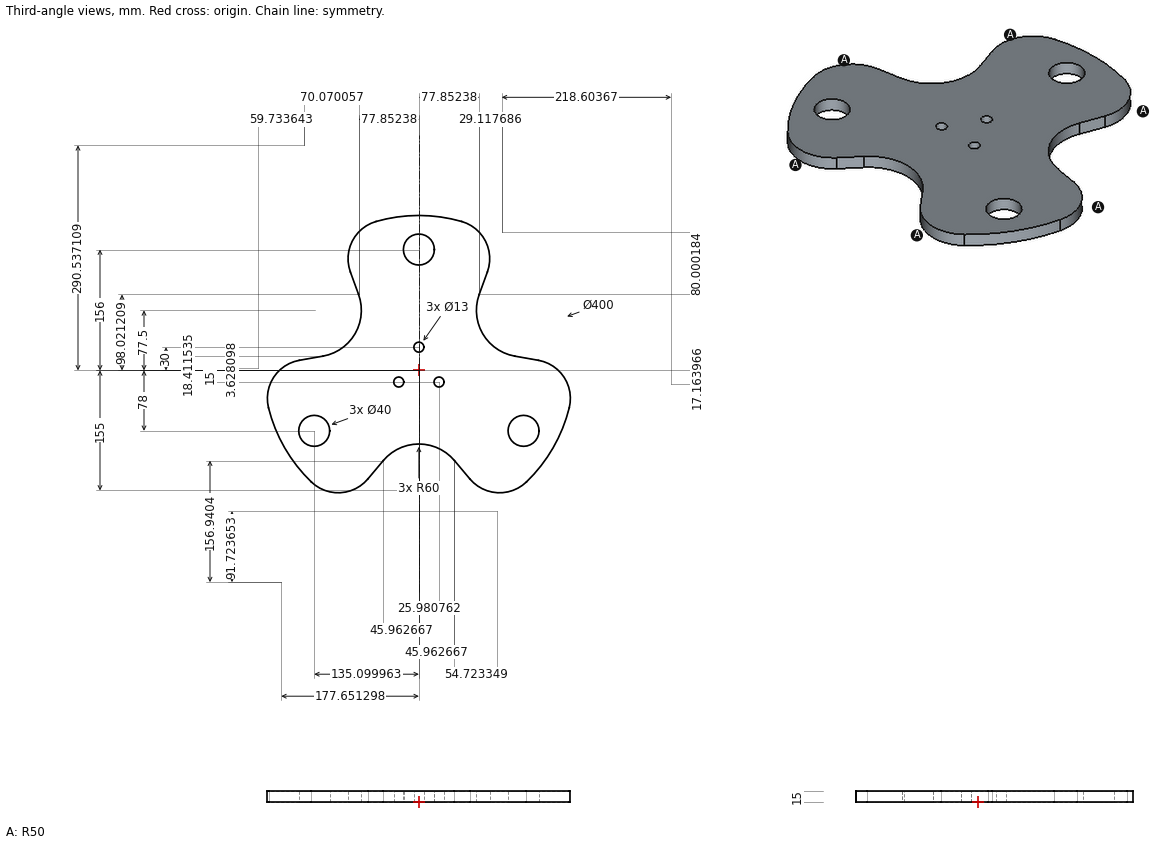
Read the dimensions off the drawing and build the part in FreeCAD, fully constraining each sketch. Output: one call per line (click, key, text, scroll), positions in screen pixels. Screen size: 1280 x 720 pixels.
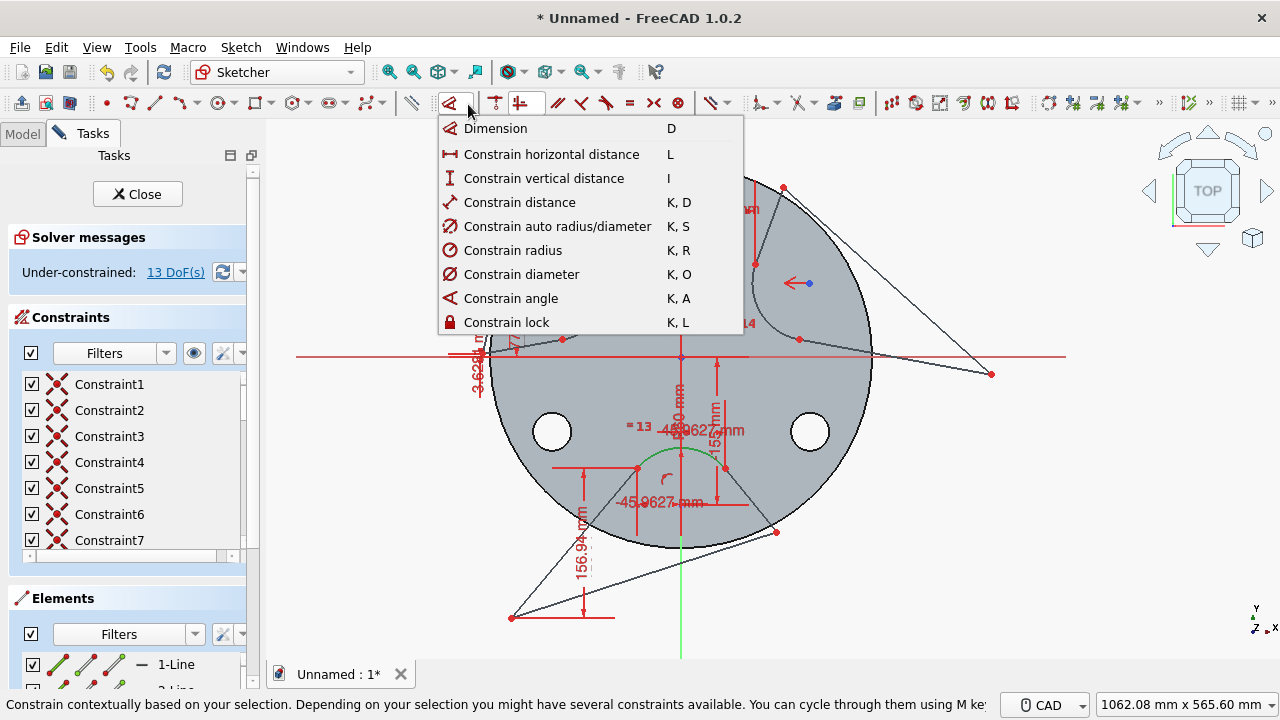
click(591, 178)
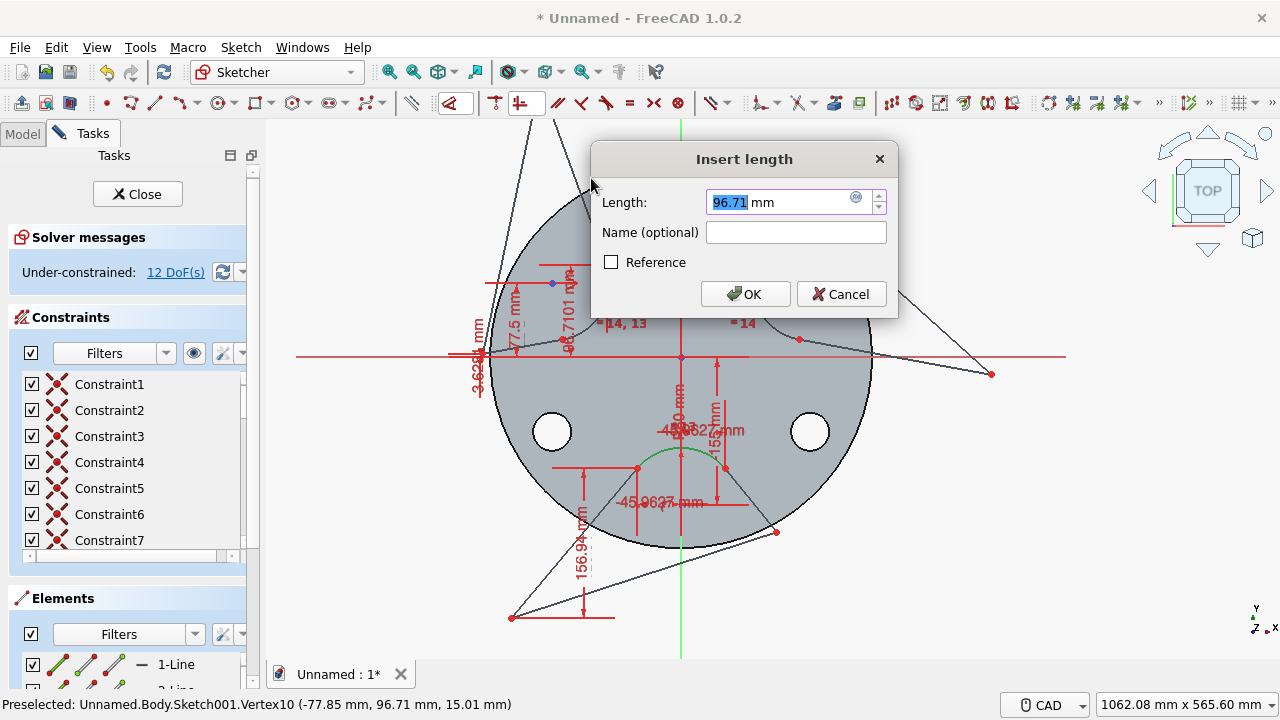
text(98.021209)
key(Return)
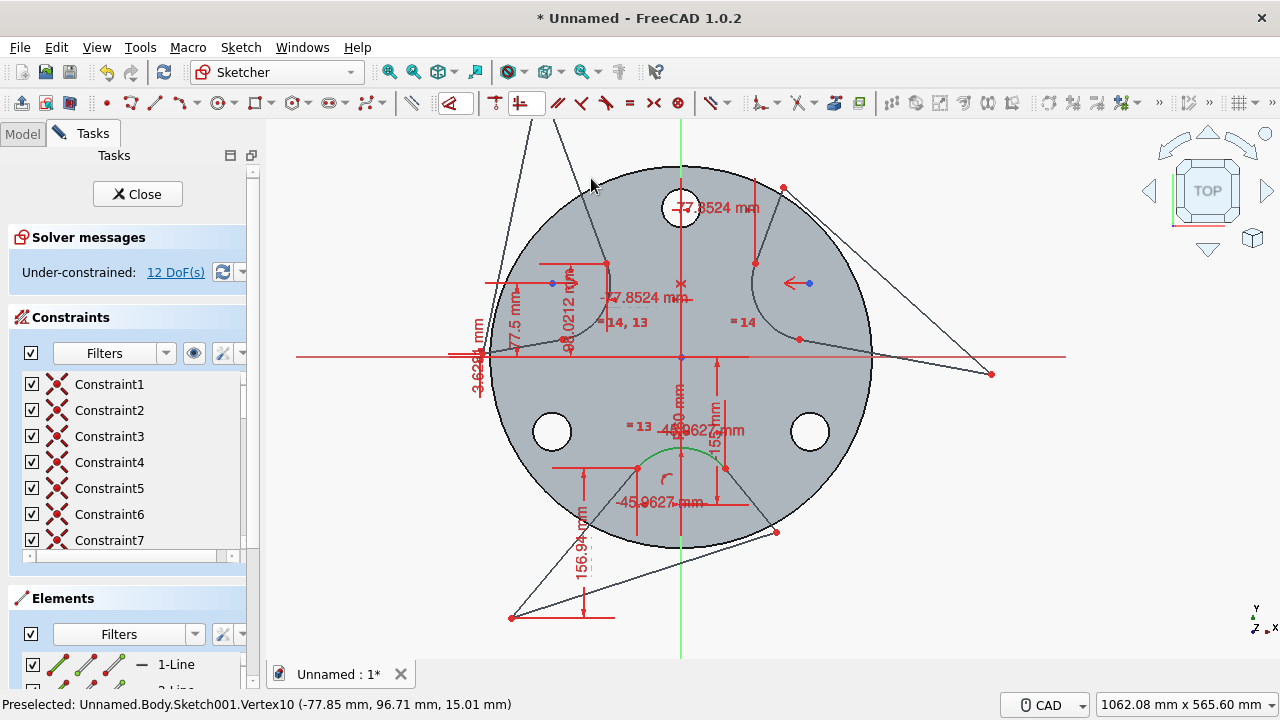
scroll(563, 340, up, 5)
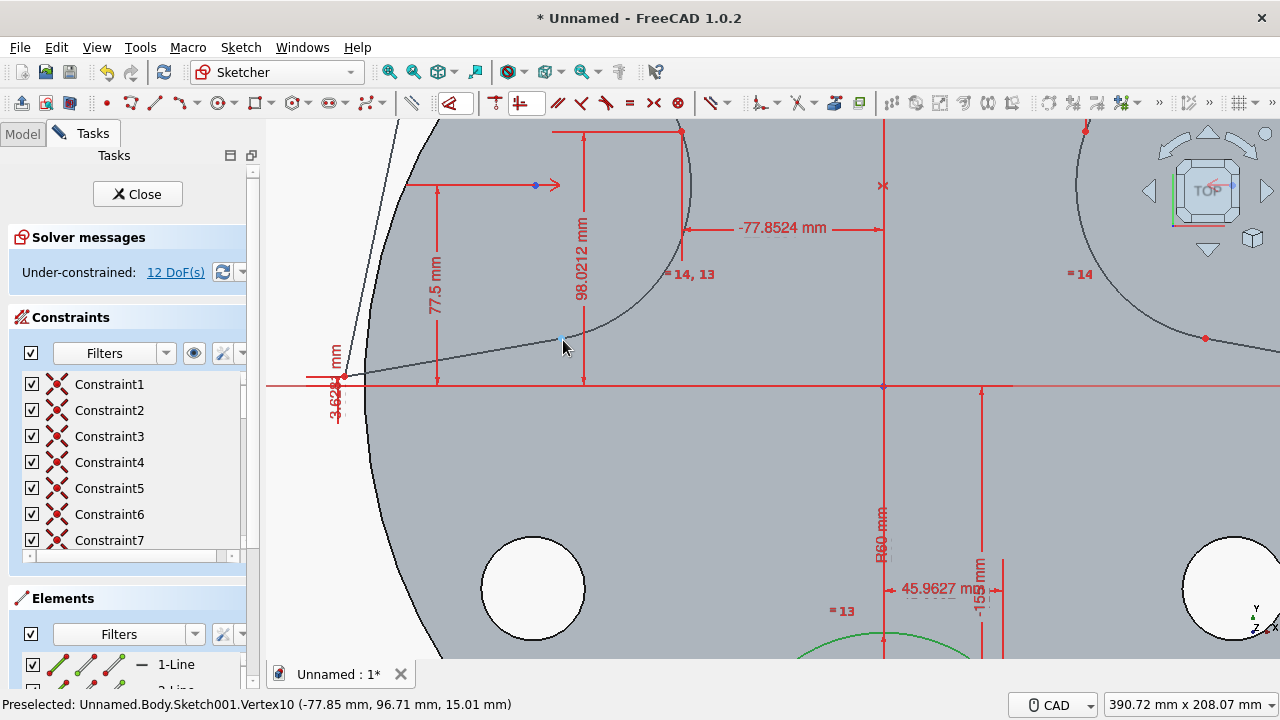
click(562, 339)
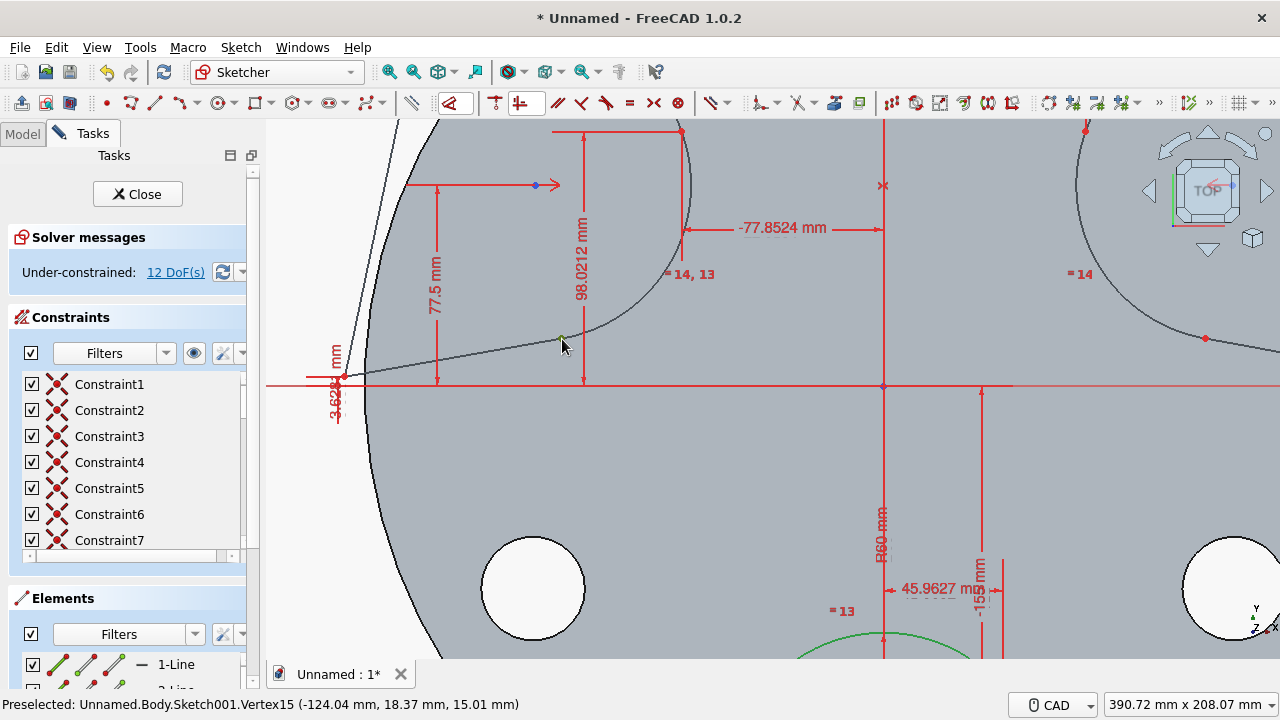
key(i)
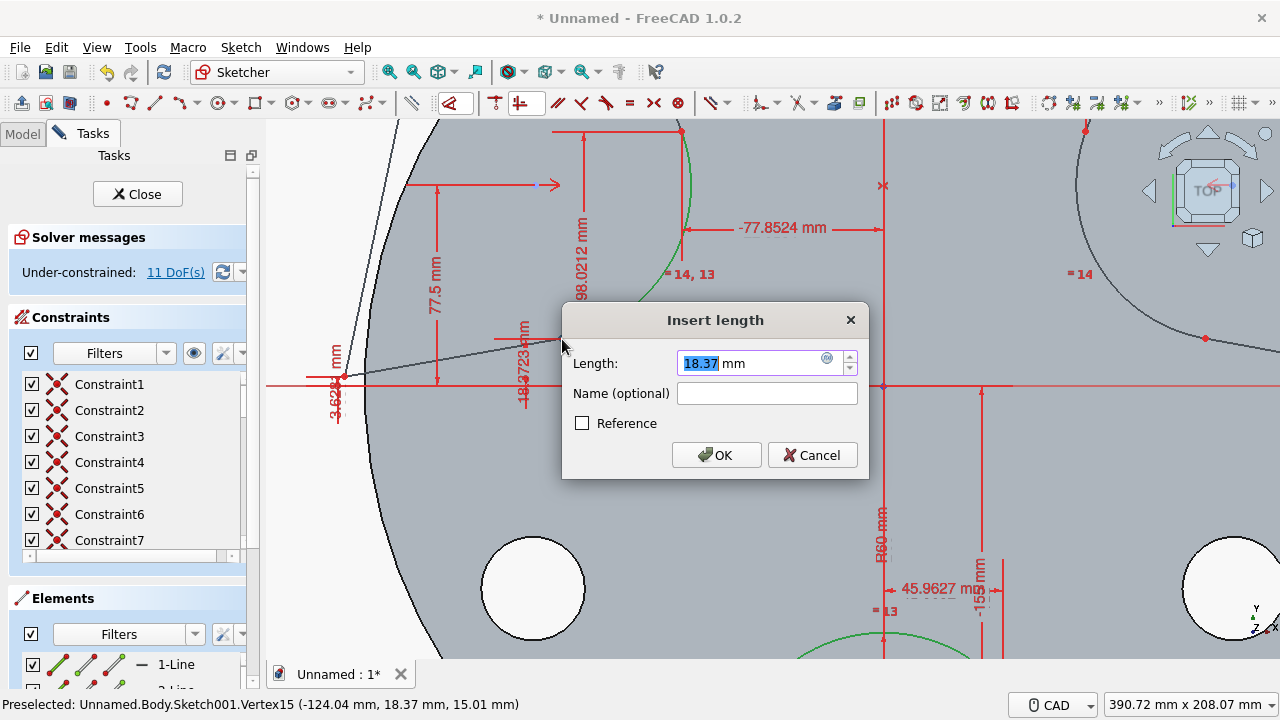
text(18.411535)
key(Return)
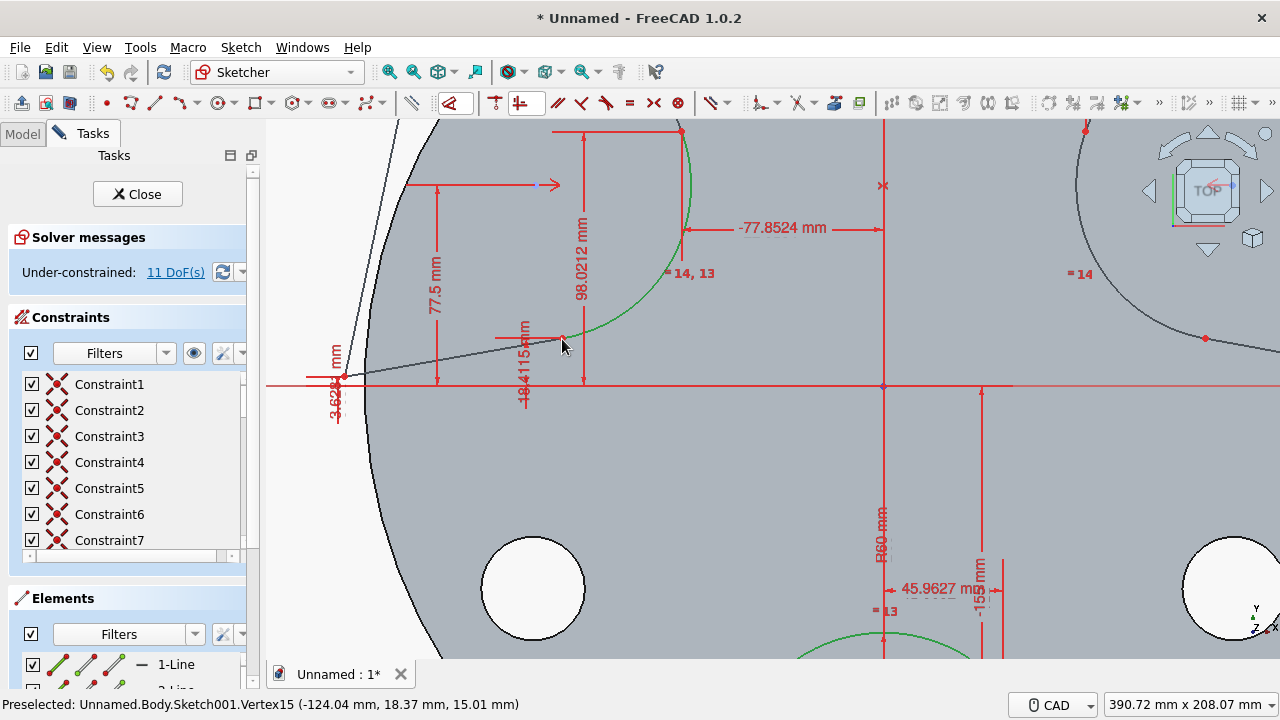
scroll(596, 397, down, 7)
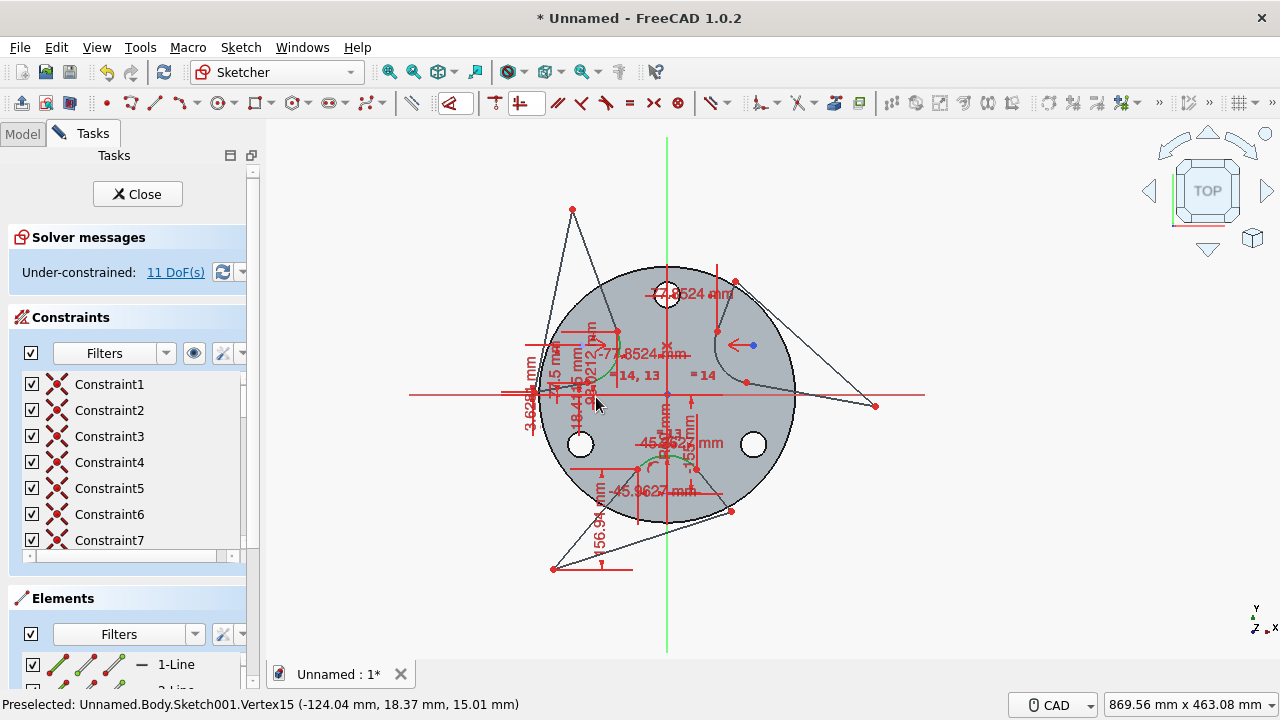
scroll(747, 383, up, 7)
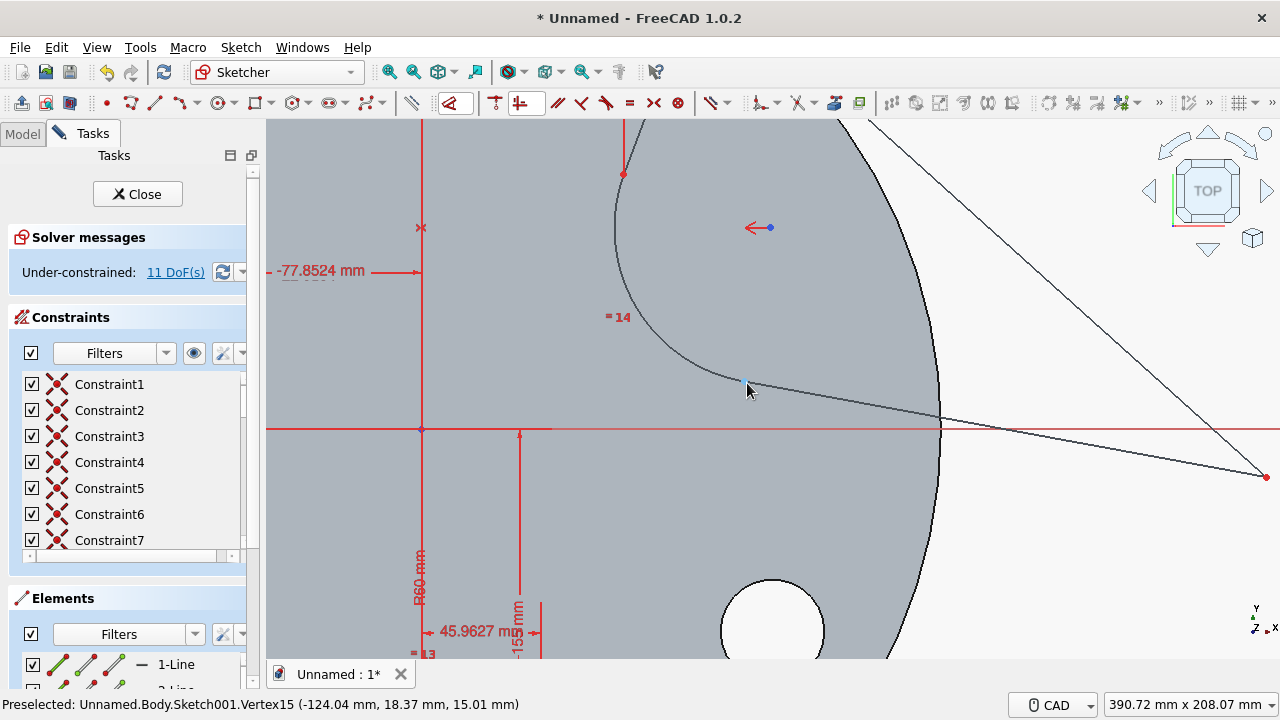
click(744, 381)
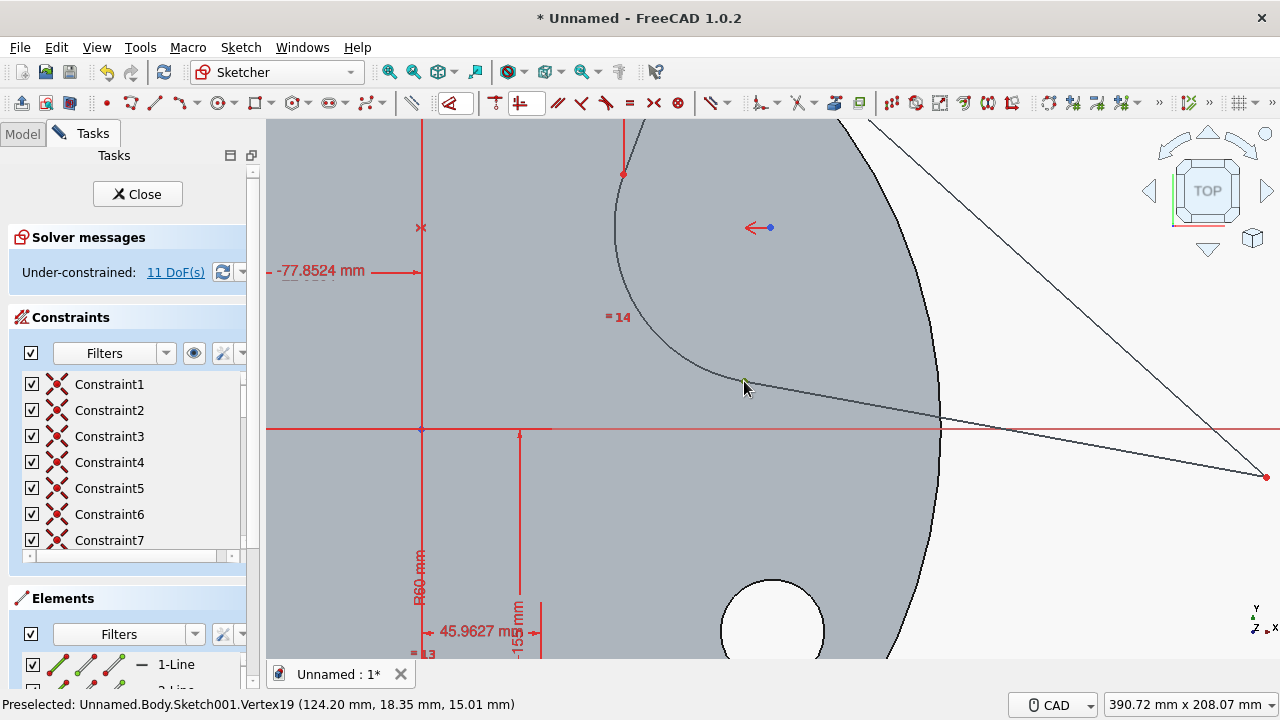
key(i)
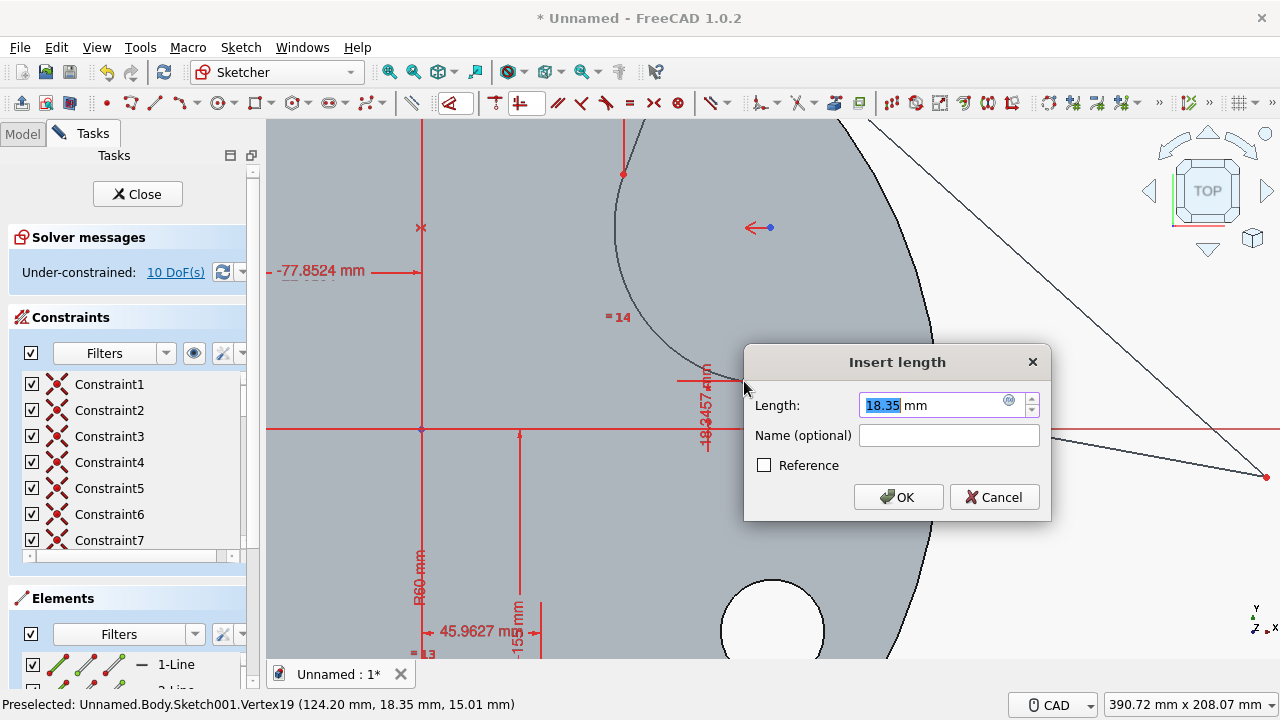
text(18.411535)
key(Return)